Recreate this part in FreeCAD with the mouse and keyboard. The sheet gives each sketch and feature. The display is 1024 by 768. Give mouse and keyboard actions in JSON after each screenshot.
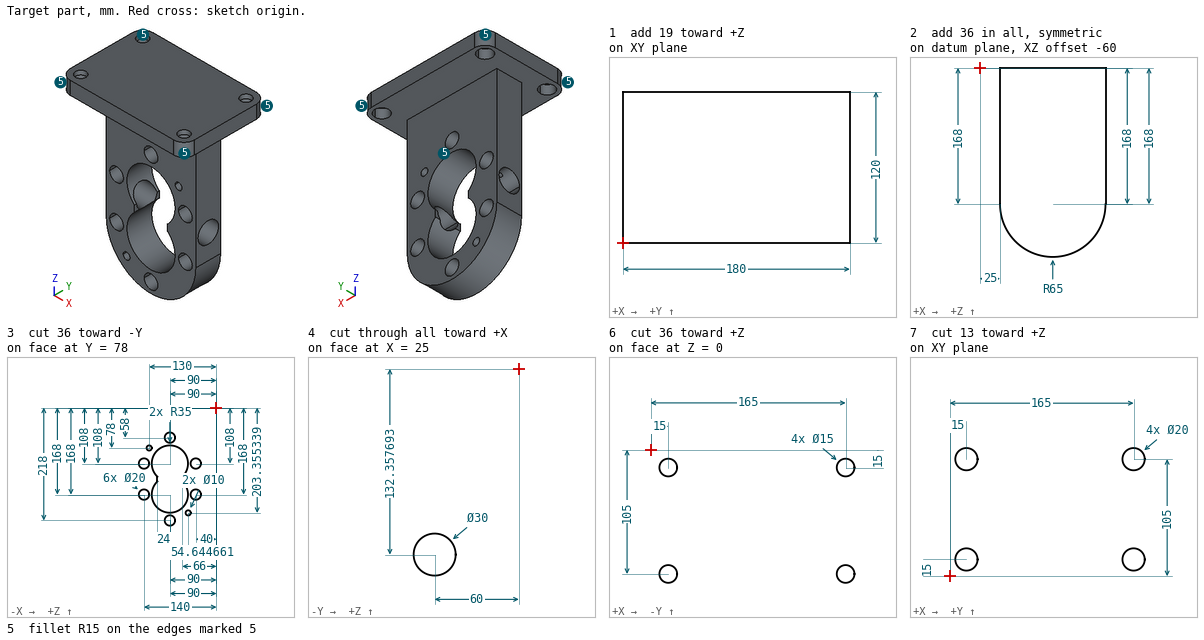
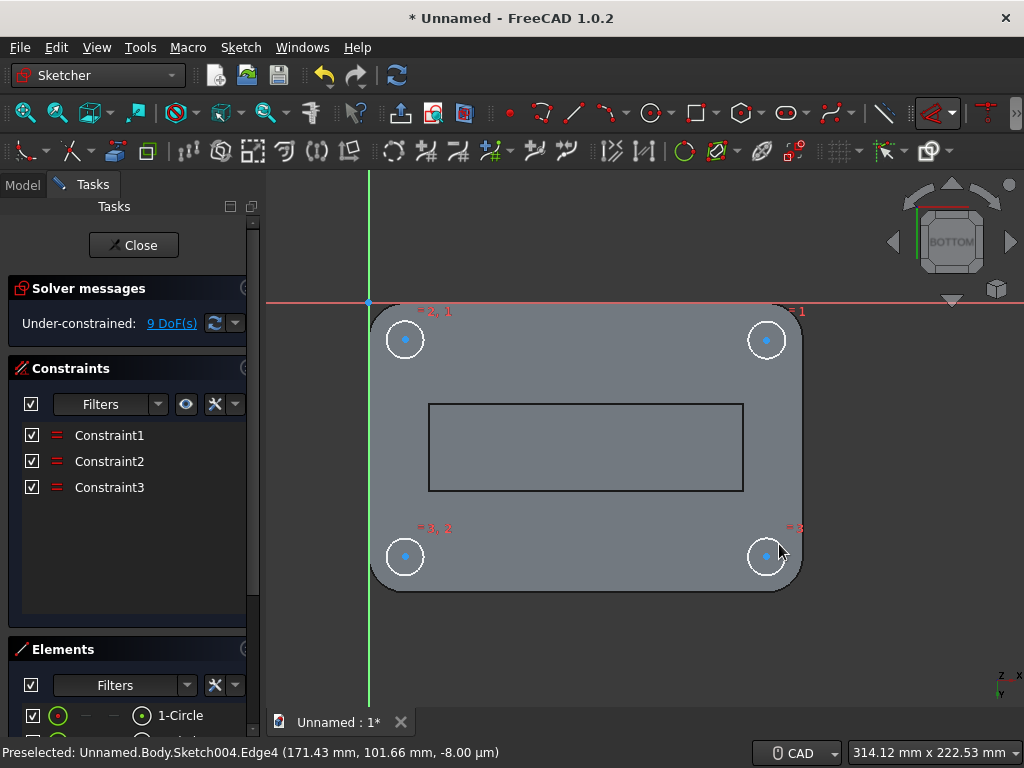
{"action": "left_click", "coordinate": [767, 340]}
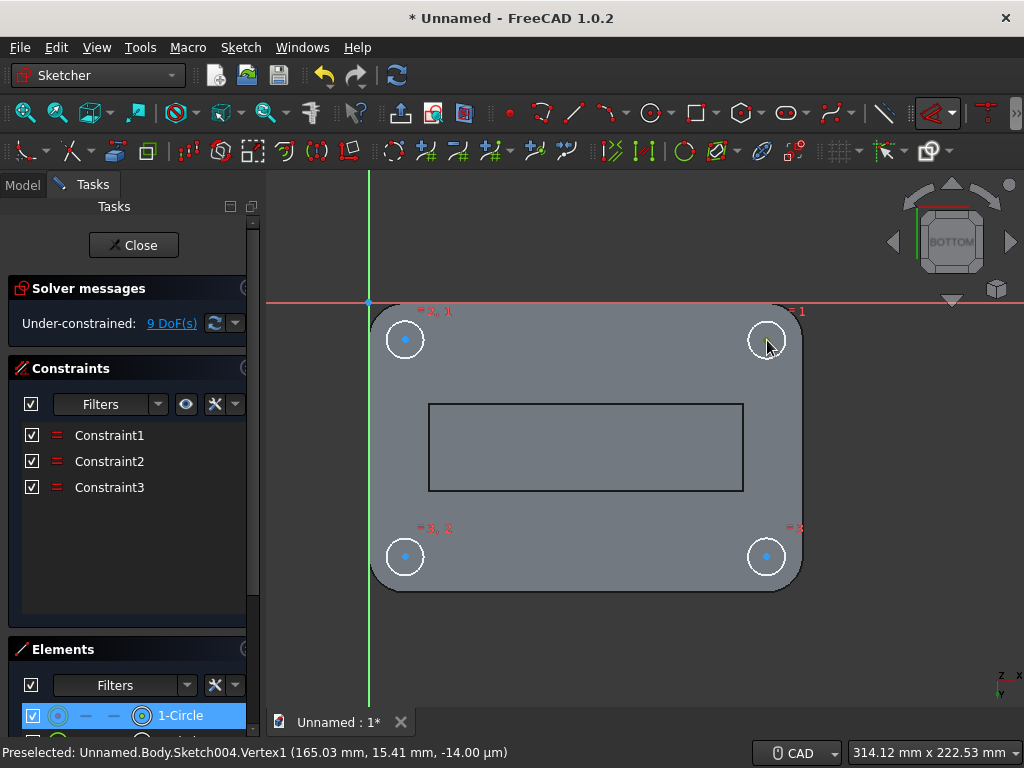
{"action": "left_click", "coordinate": [405, 340]}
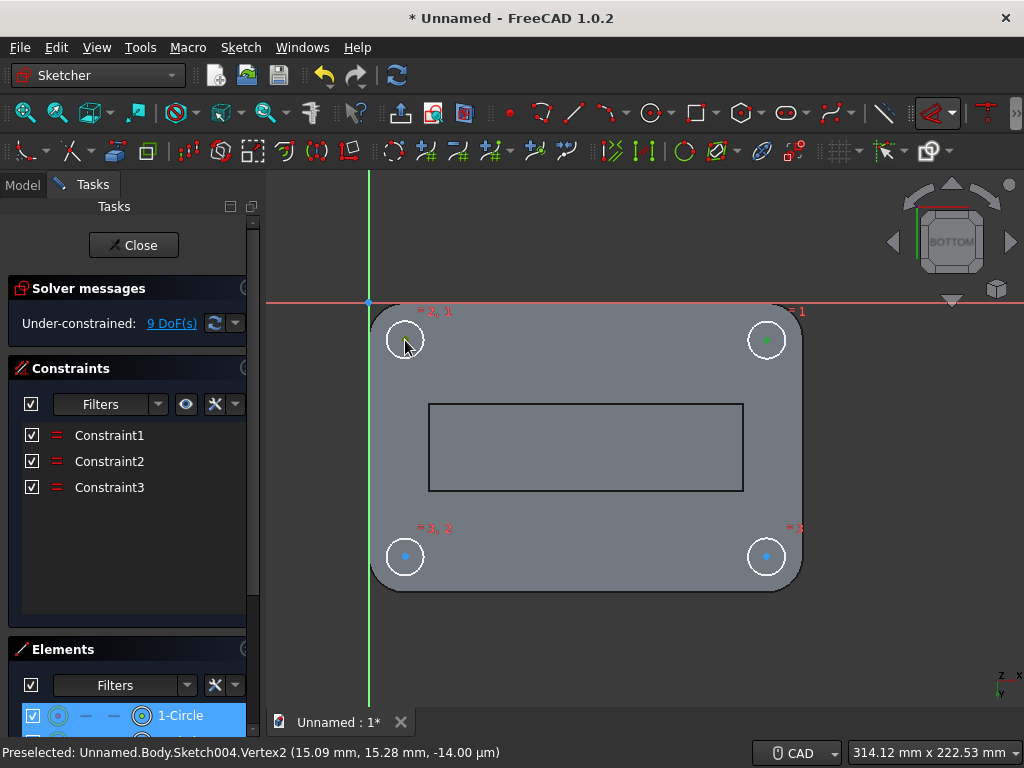
{"action": "key", "text": "h"}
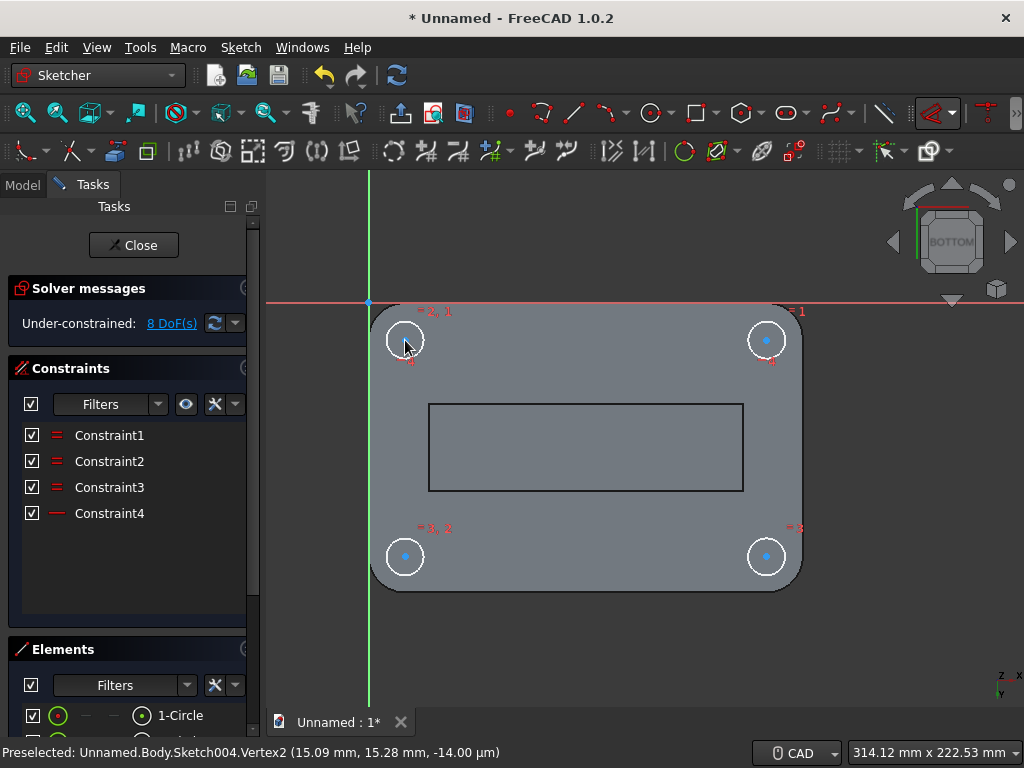
{"action": "left_click", "coordinate": [405, 340]}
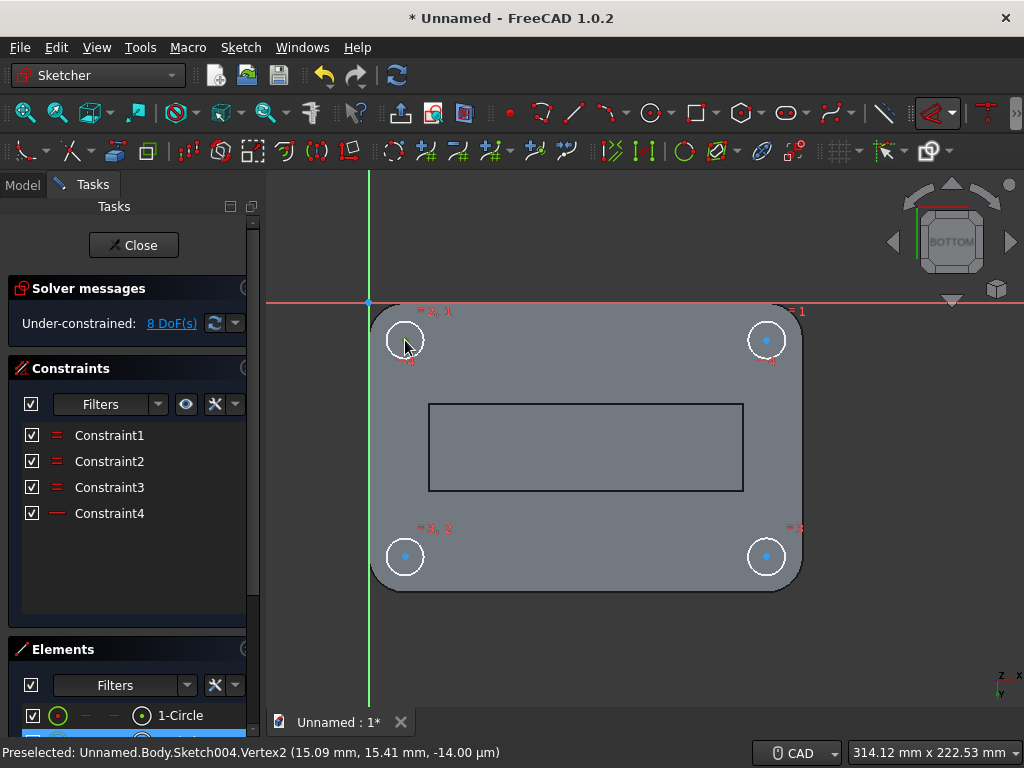
{"action": "left_click", "coordinate": [405, 557]}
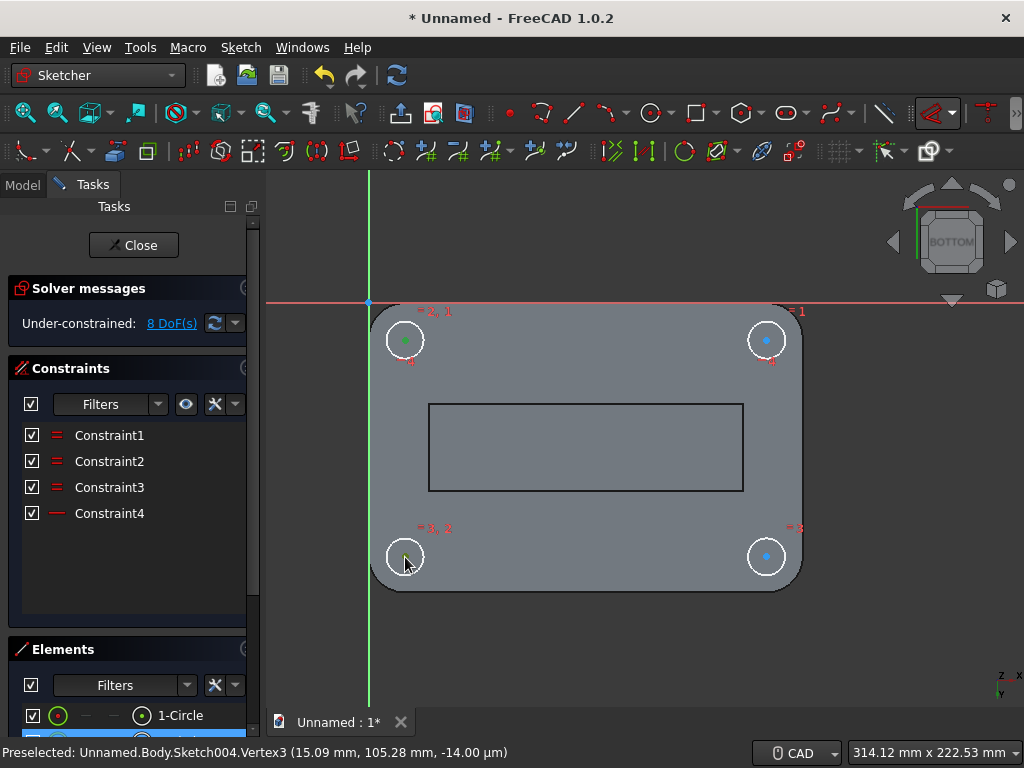
{"action": "key", "text": "v"}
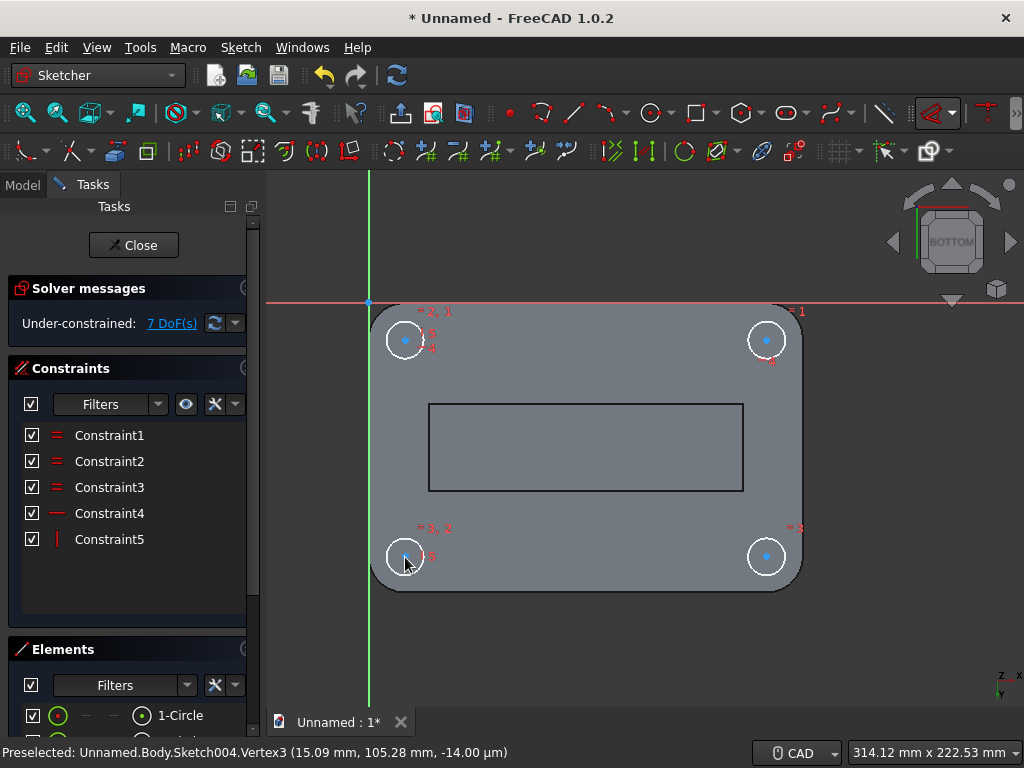
{"action": "left_click", "coordinate": [767, 340]}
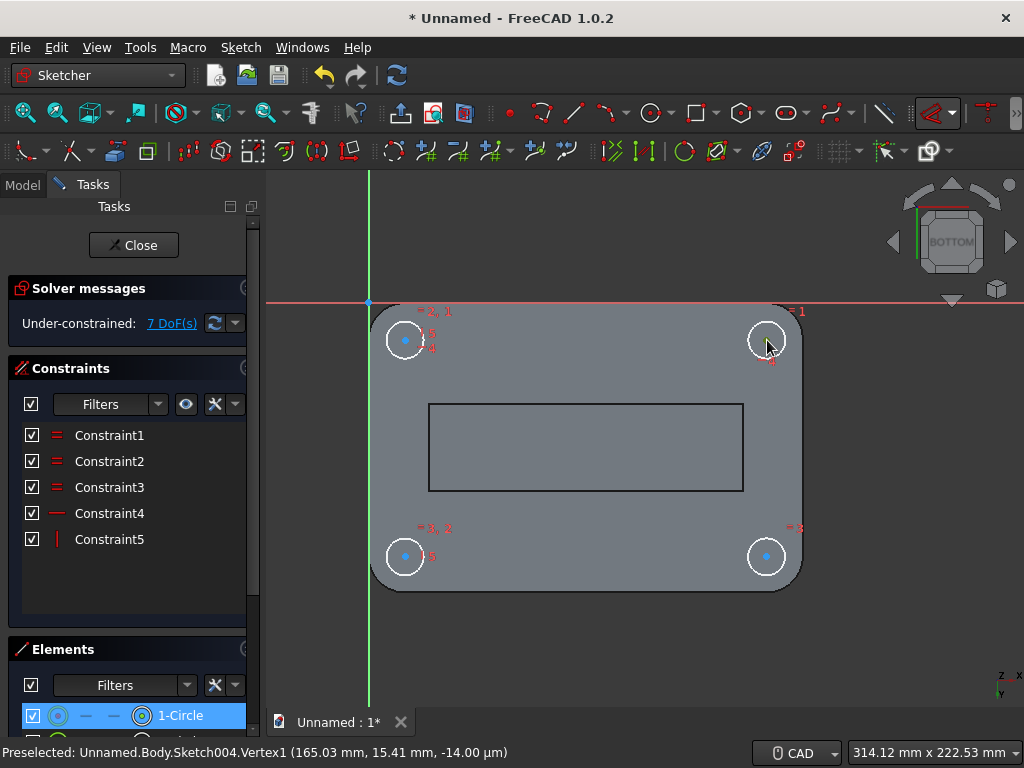
{"action": "left_click", "coordinate": [767, 557]}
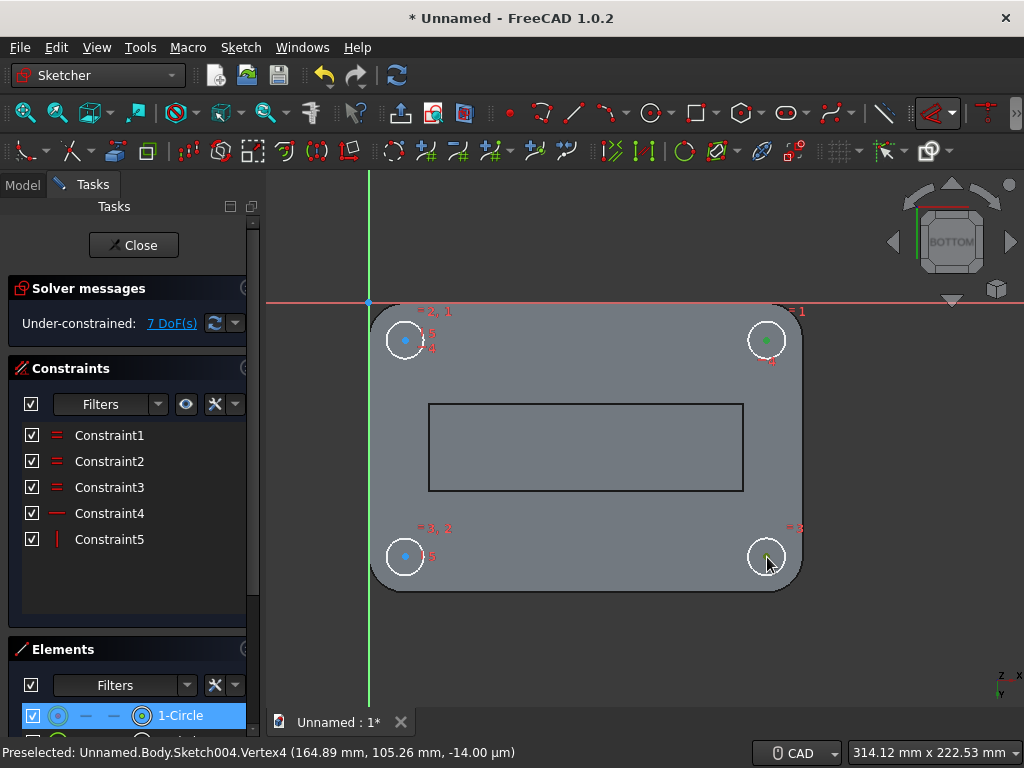
{"action": "key", "text": "v"}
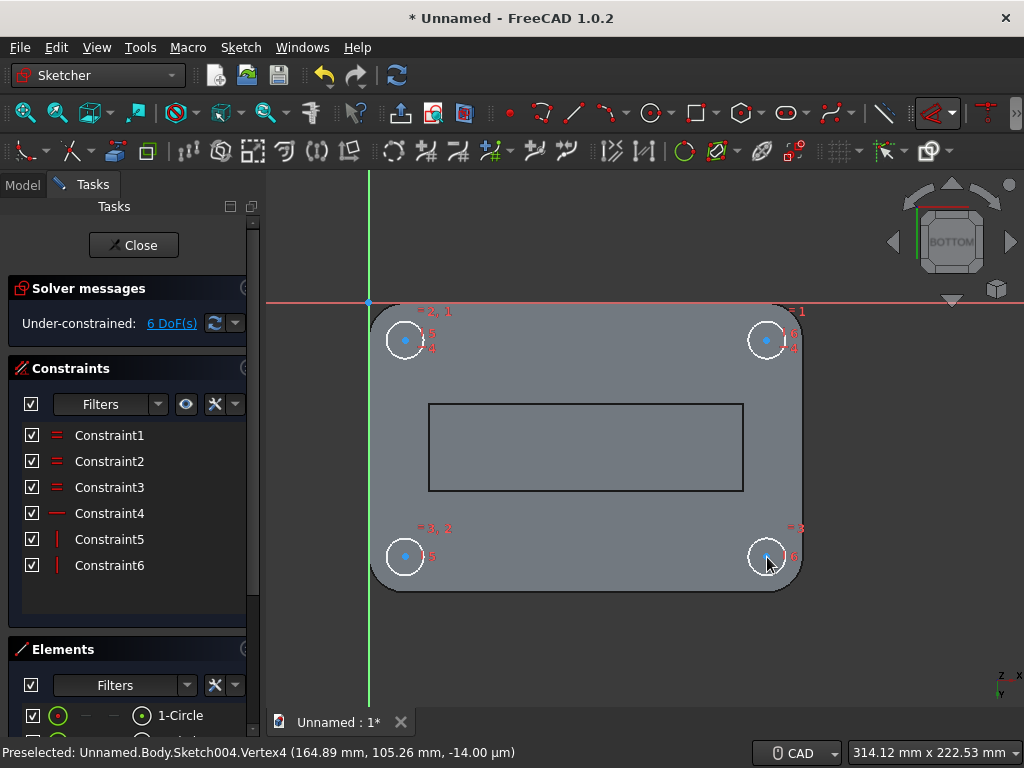
{"action": "left_click", "coordinate": [405, 557]}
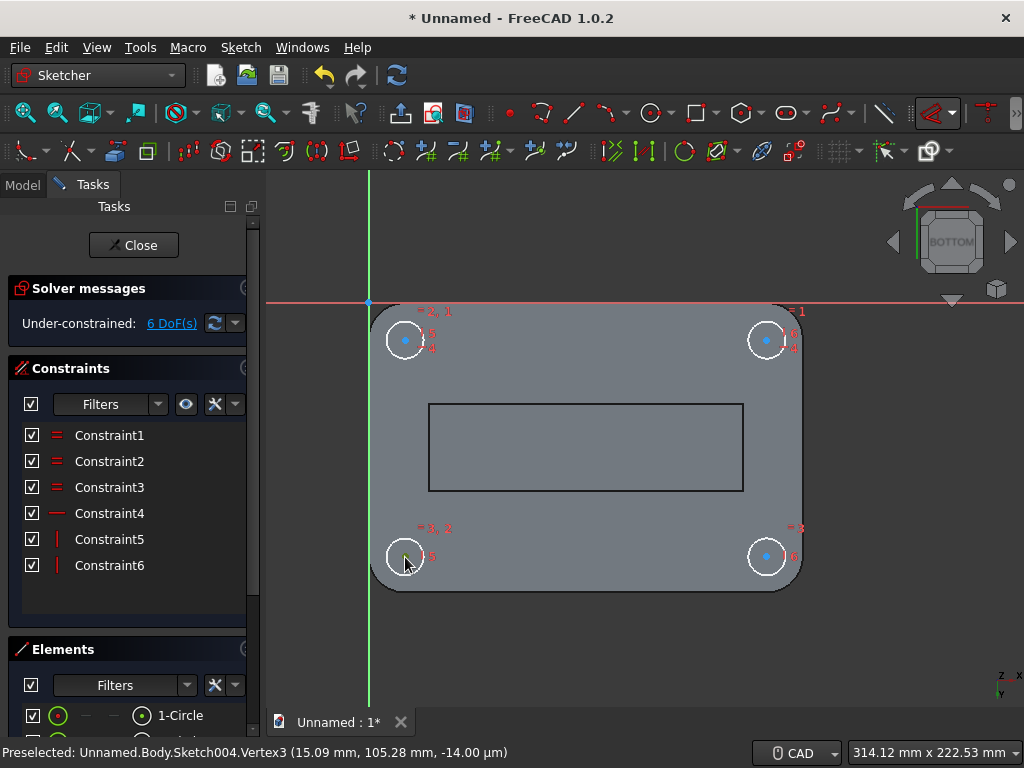
{"action": "left_click", "coordinate": [767, 557]}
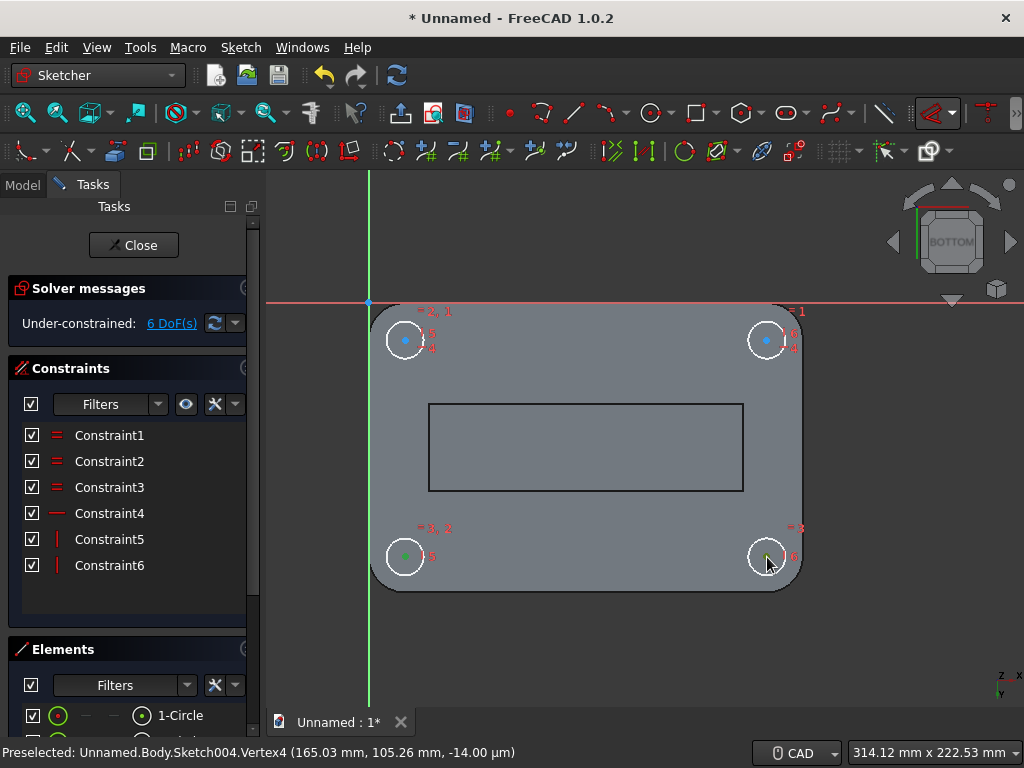
{"action": "key", "text": "h"}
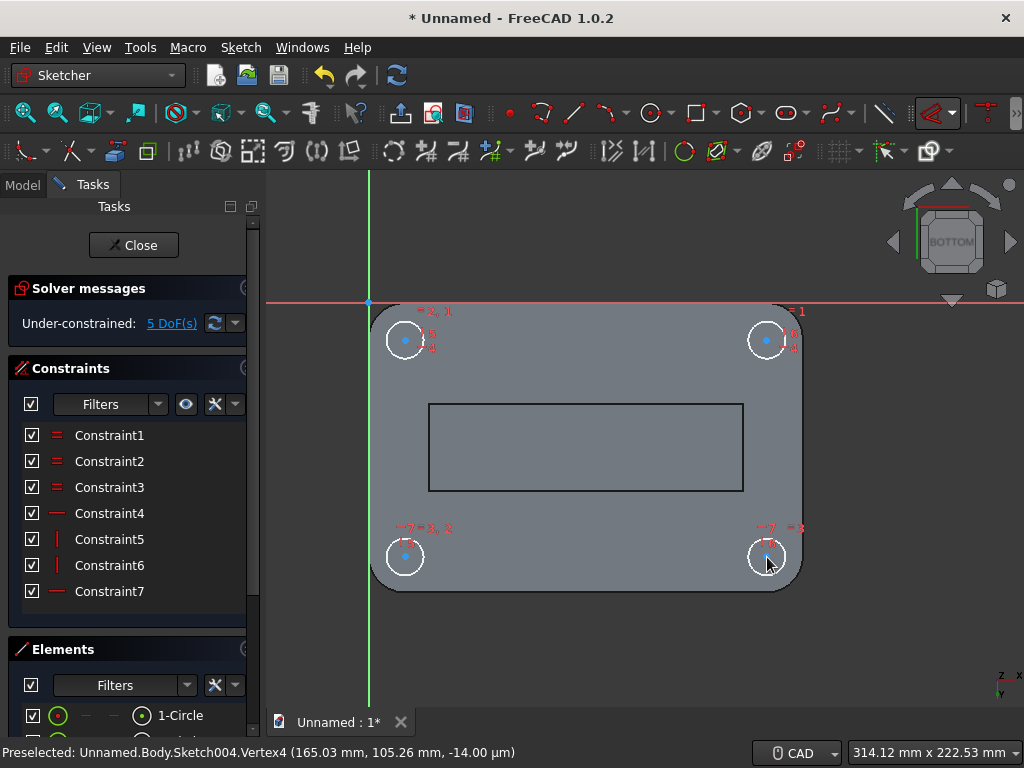
{"action": "left_click", "coordinate": [754, 327]}